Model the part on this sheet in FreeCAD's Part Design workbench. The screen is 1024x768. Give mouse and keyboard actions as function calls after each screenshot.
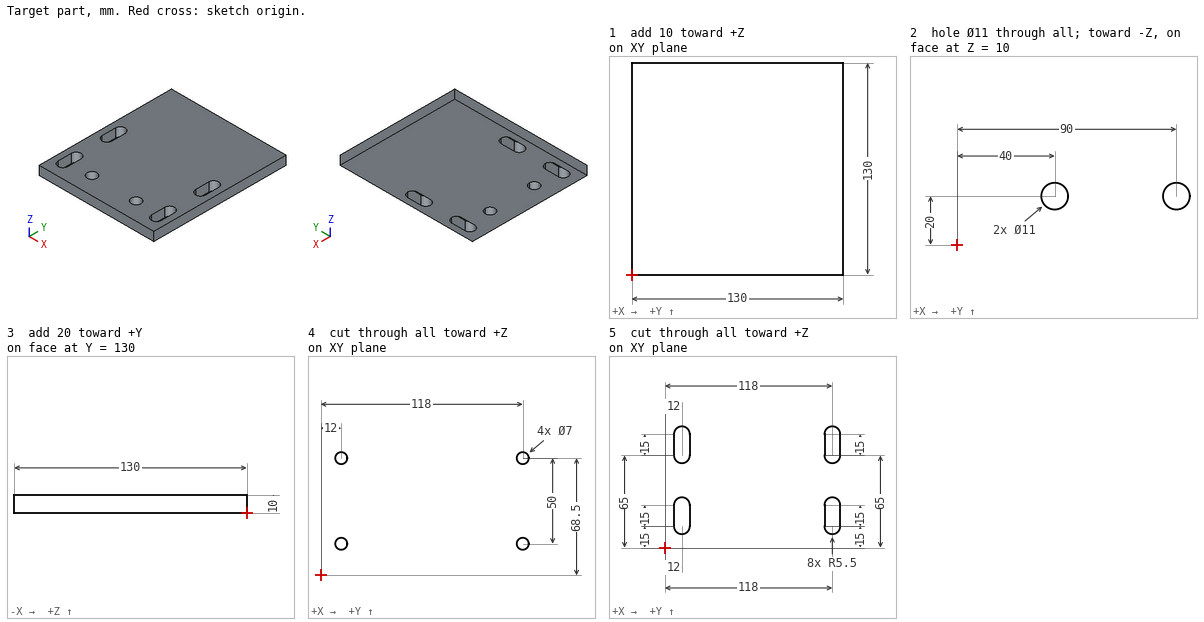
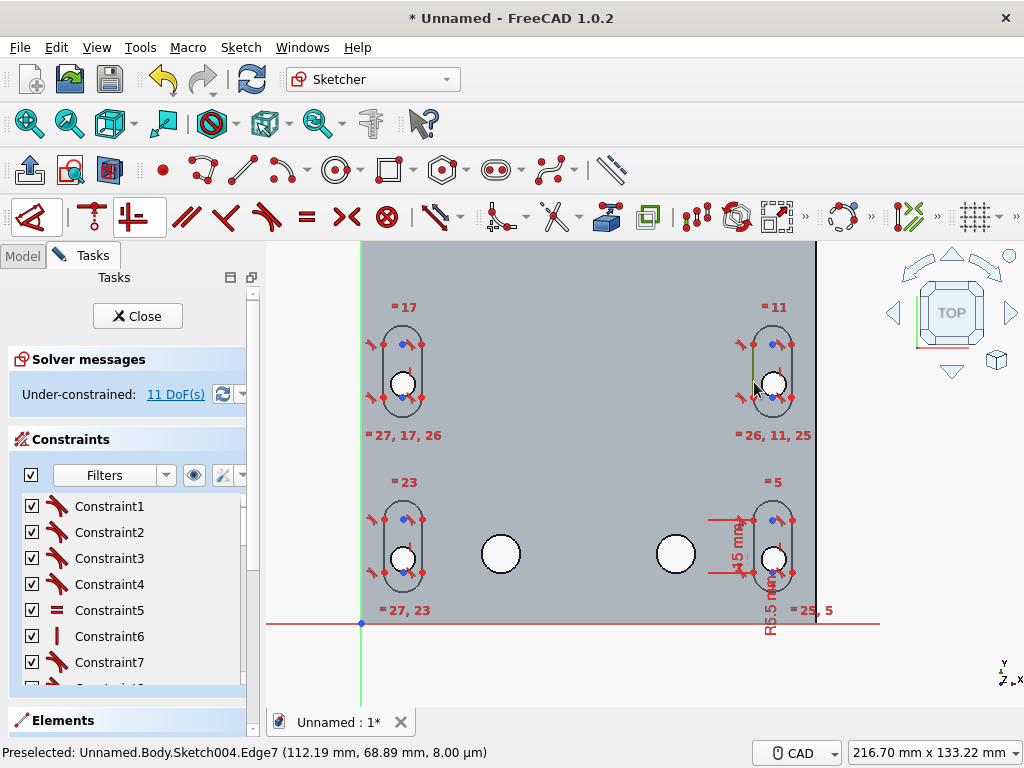
click(56, 218)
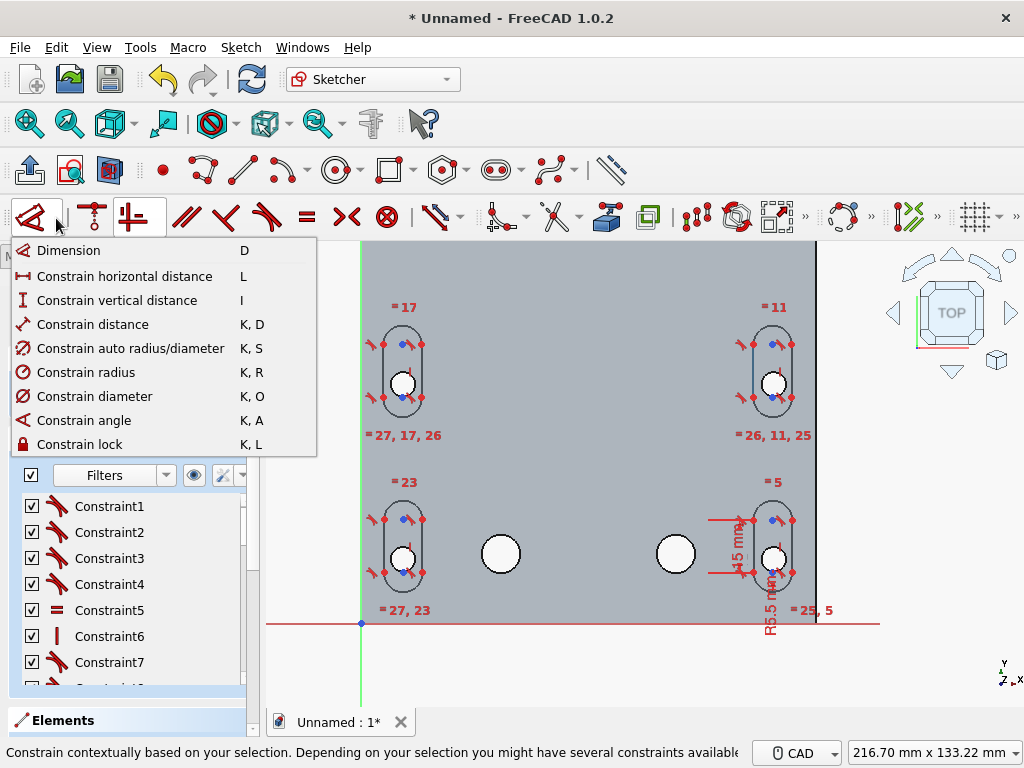
click(164, 300)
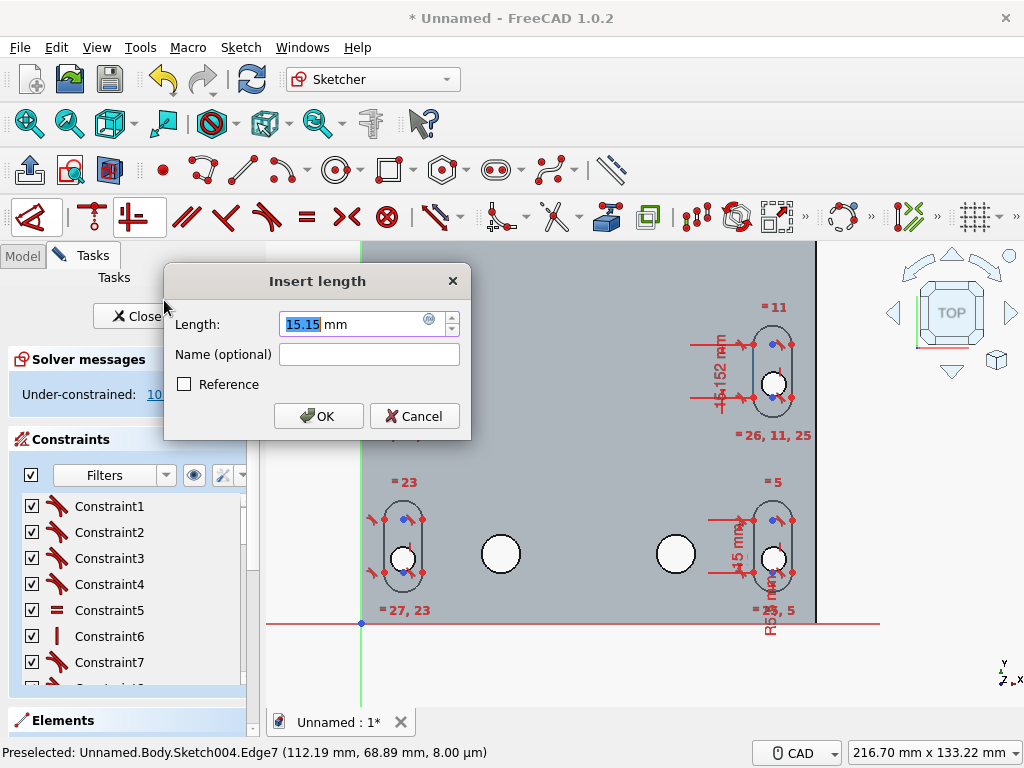
text(15)
key(Return)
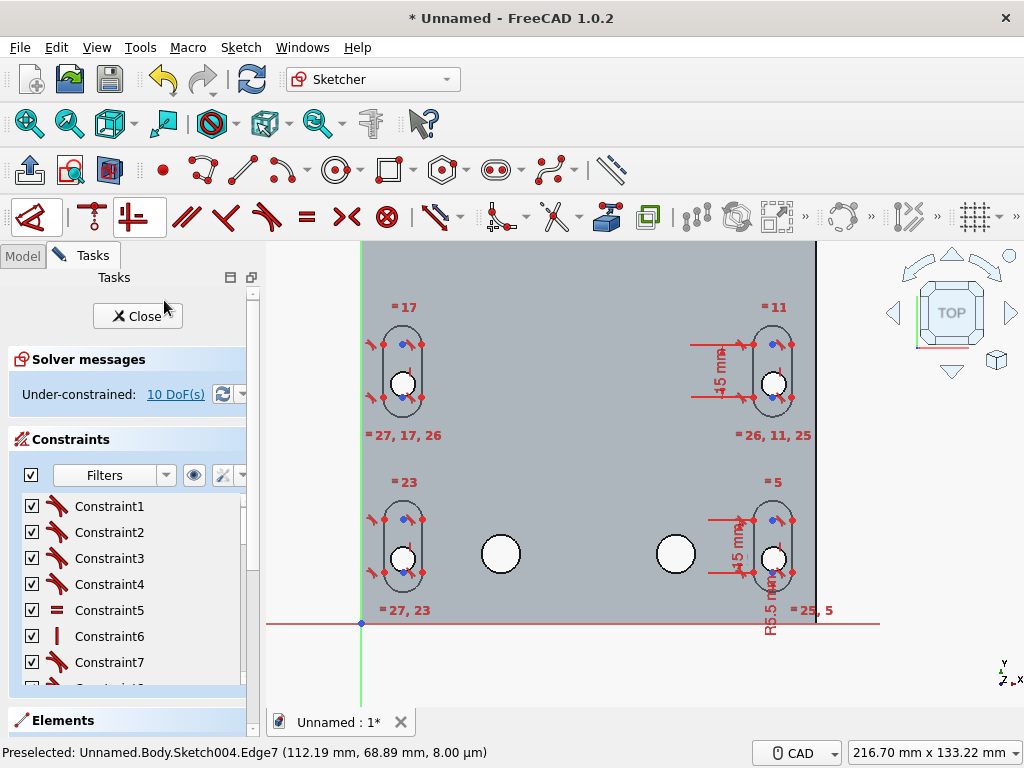
click(383, 382)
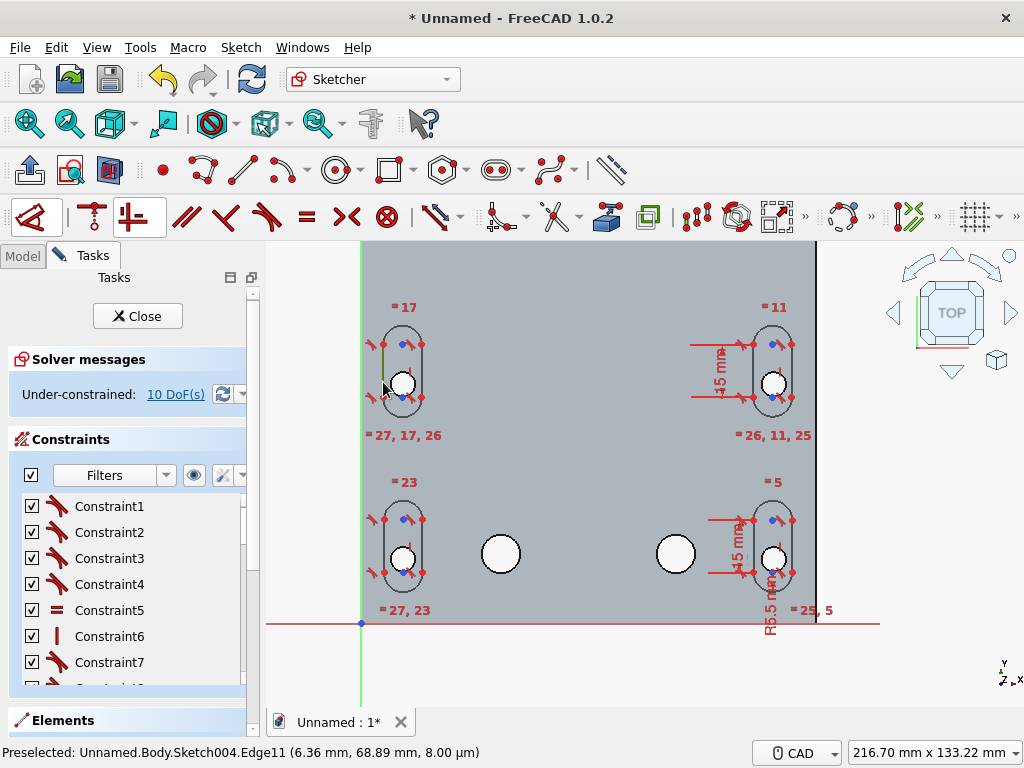
key(i)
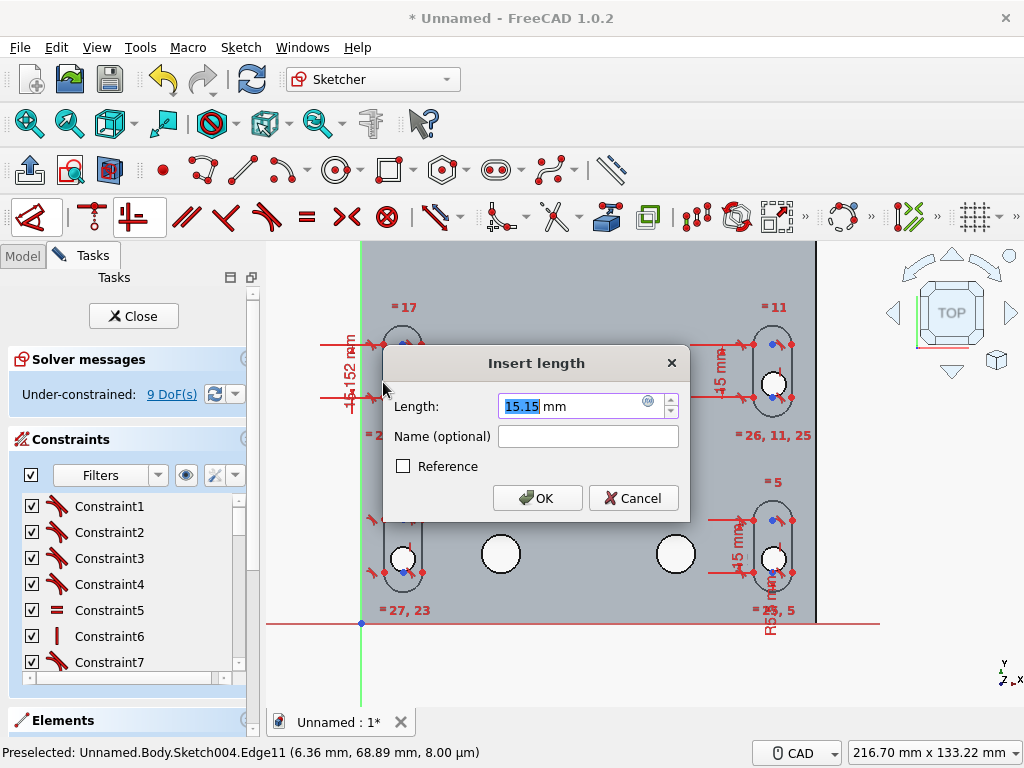
text(15)
key(Return)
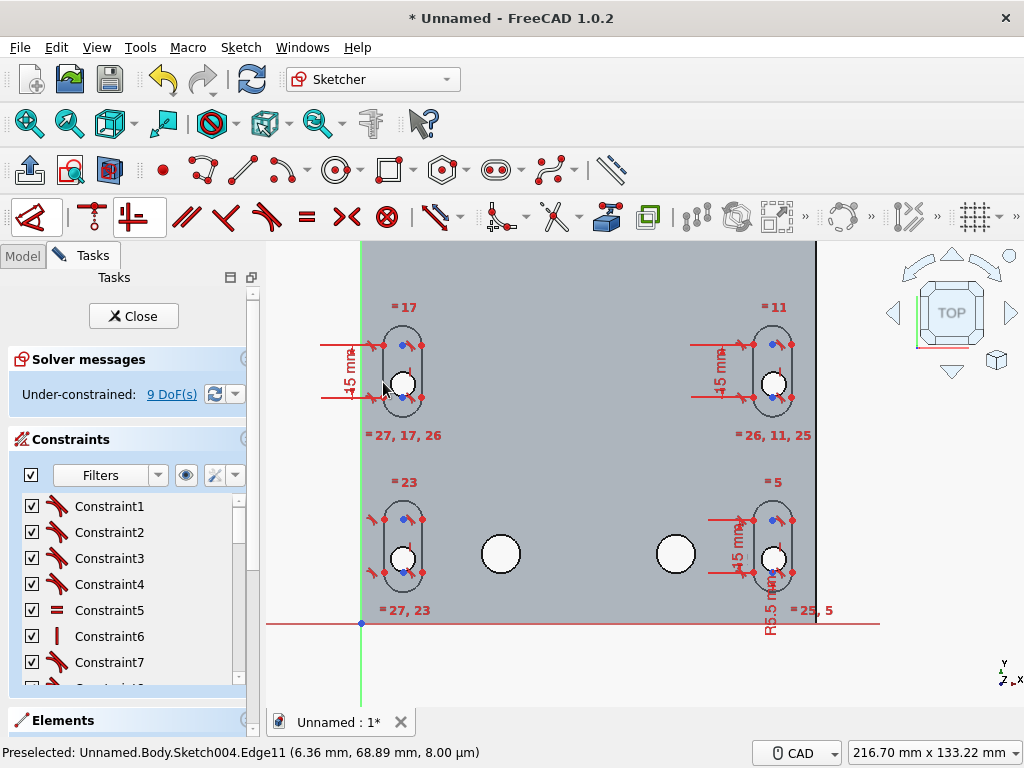
click(384, 557)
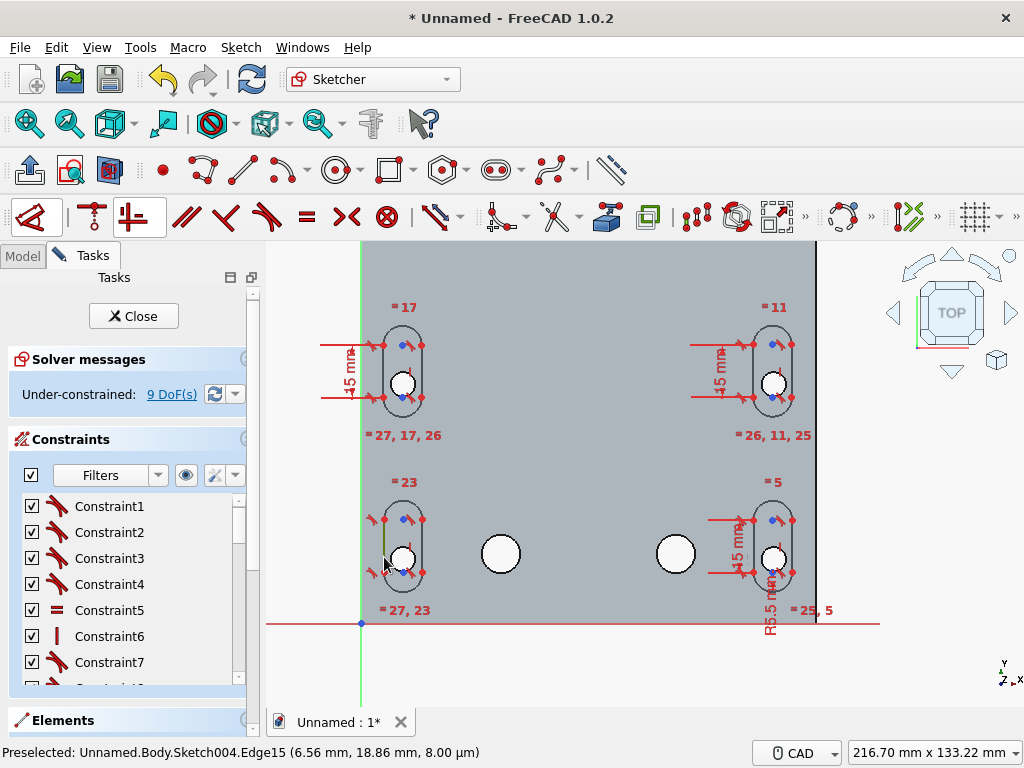
click(56, 218)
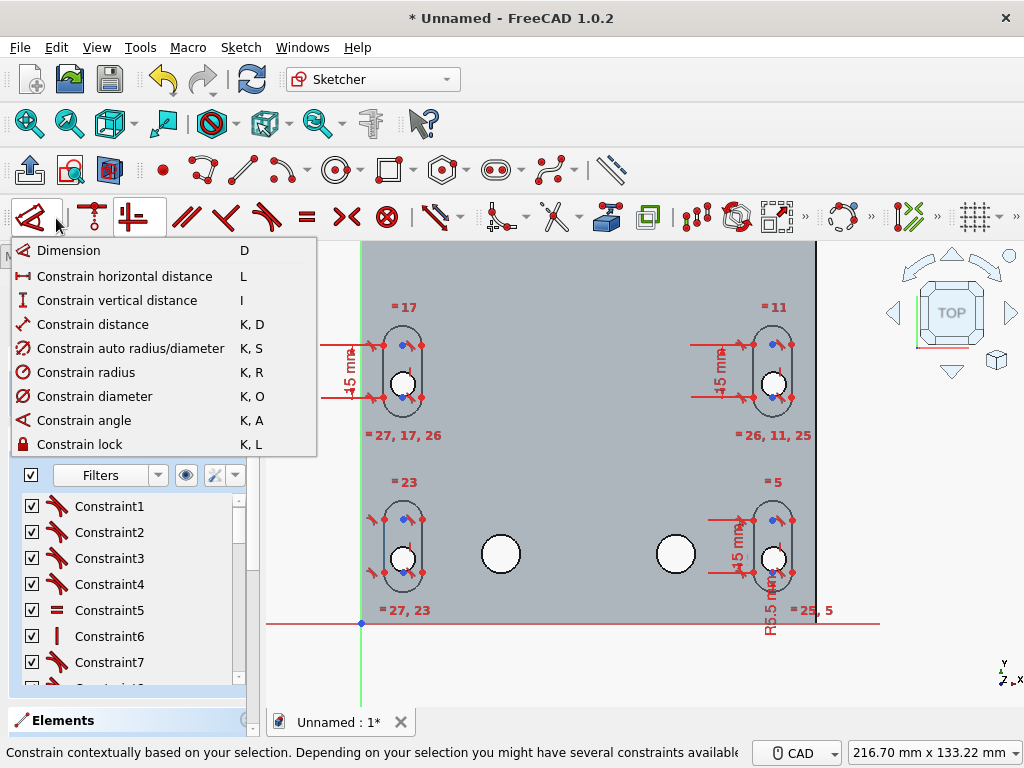
click(164, 300)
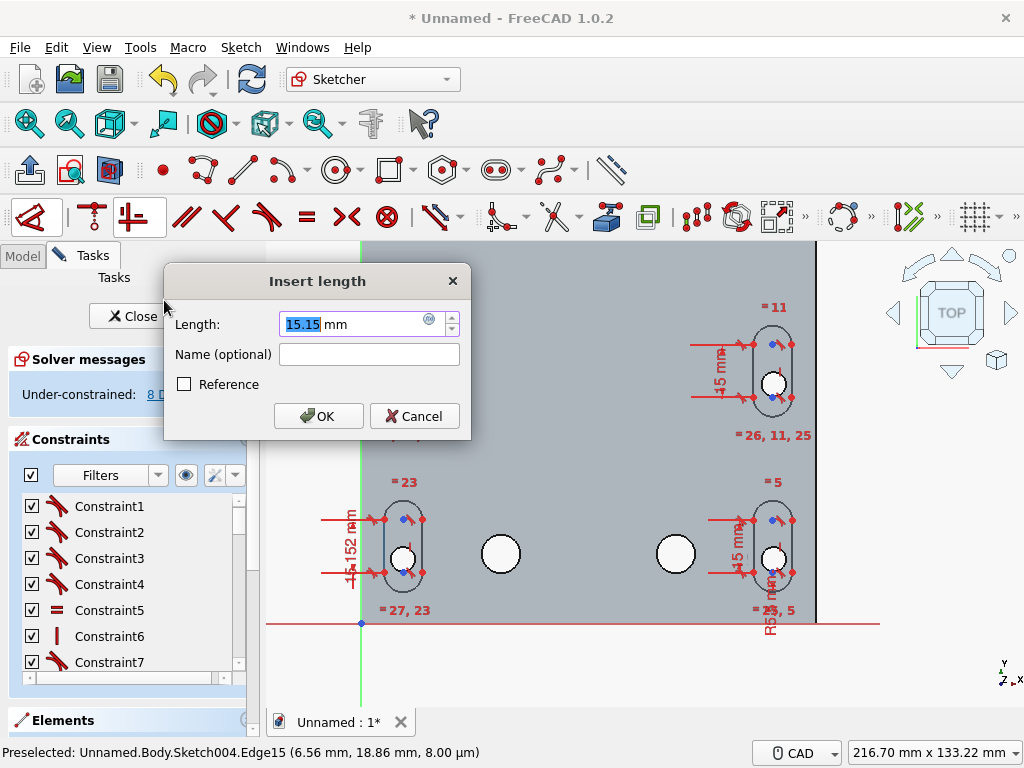
text(15)
key(Return)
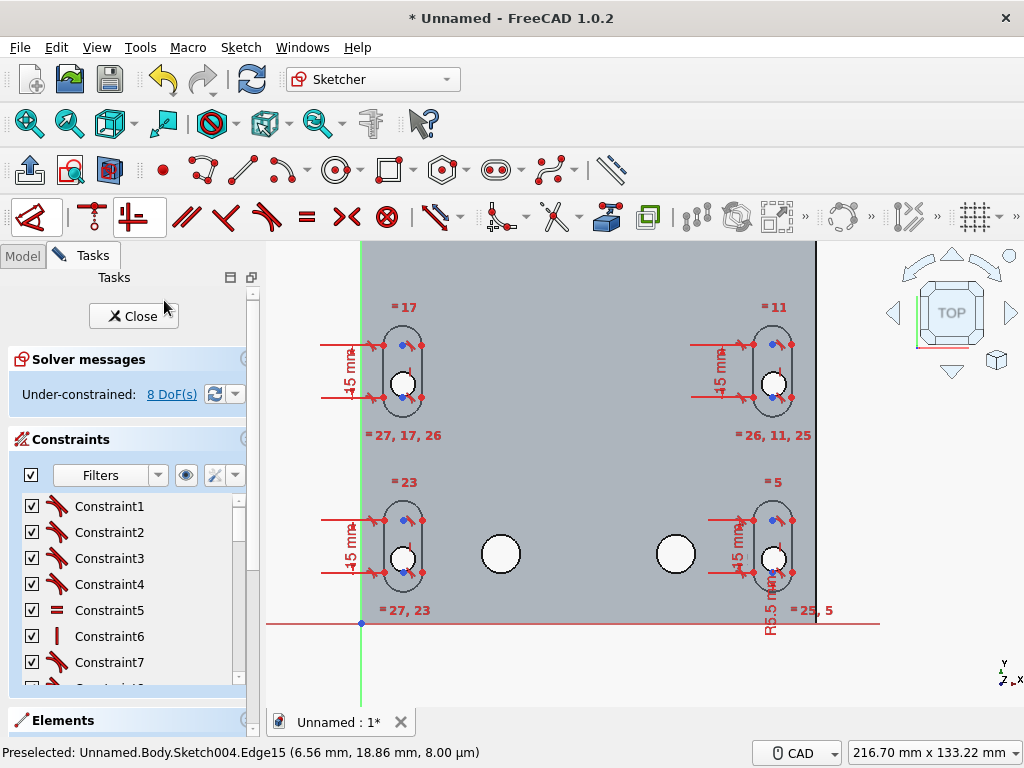
click(754, 573)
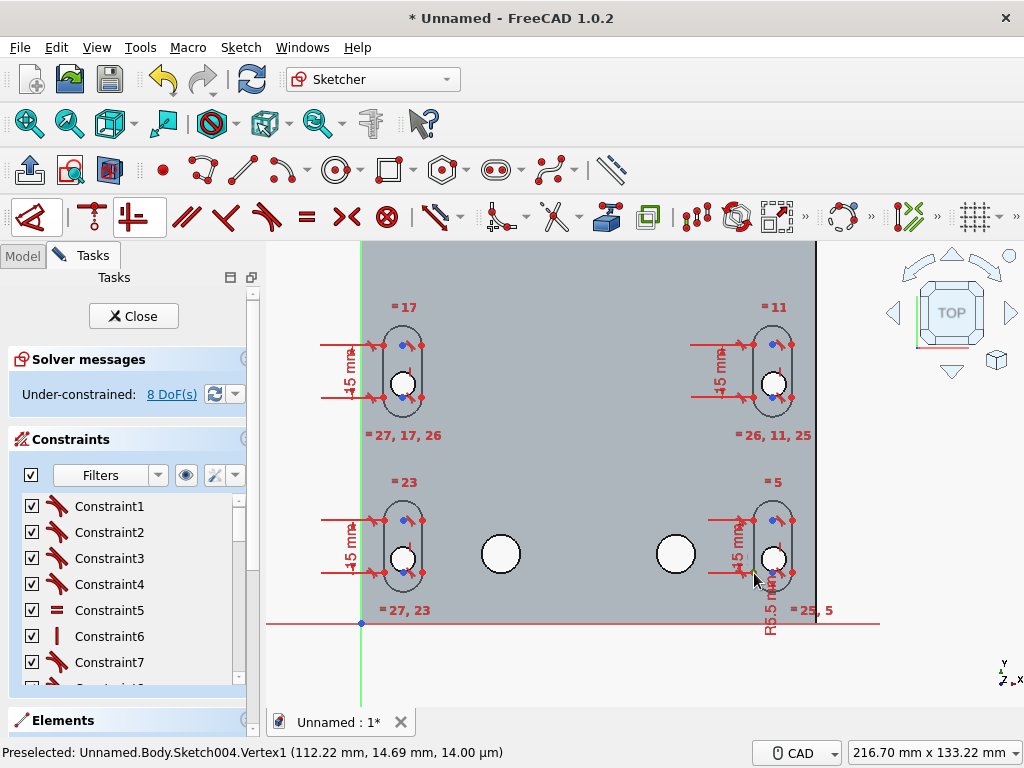
key(i)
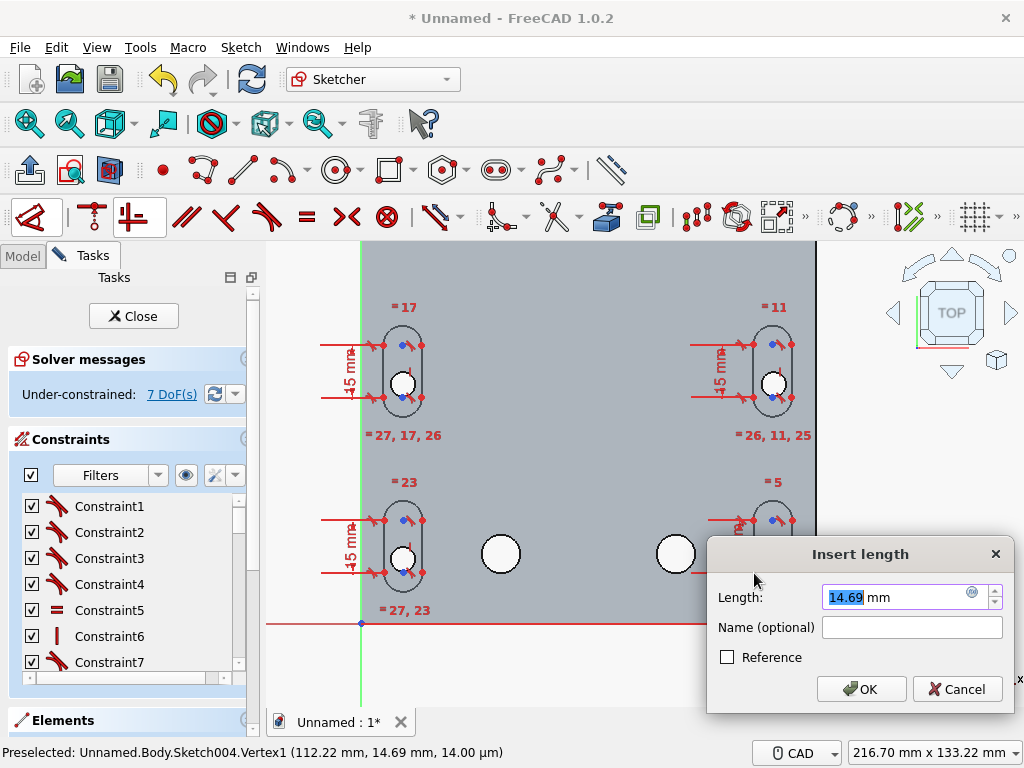
text(15)
key(Return)